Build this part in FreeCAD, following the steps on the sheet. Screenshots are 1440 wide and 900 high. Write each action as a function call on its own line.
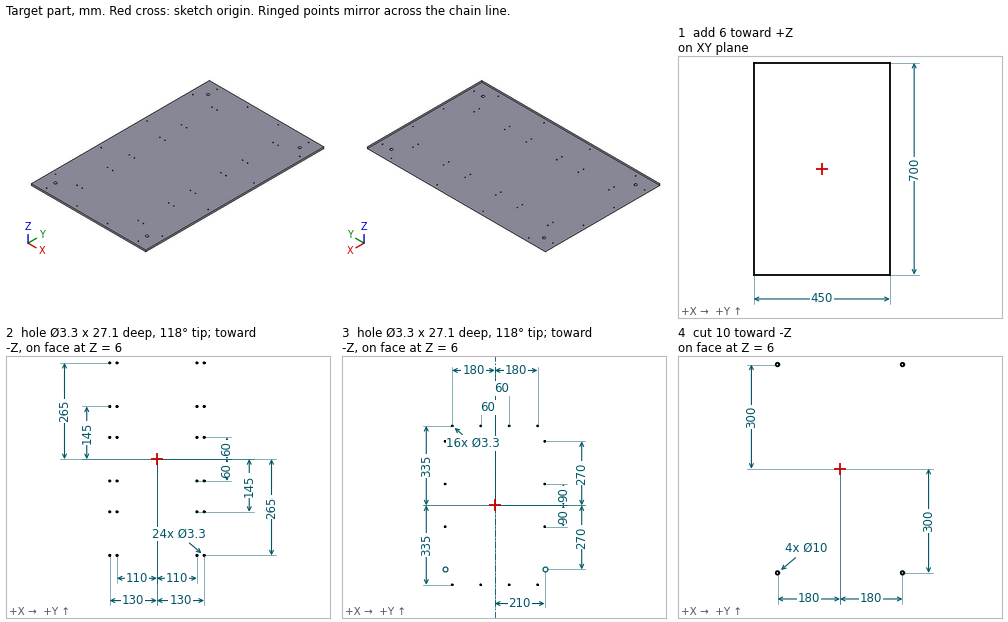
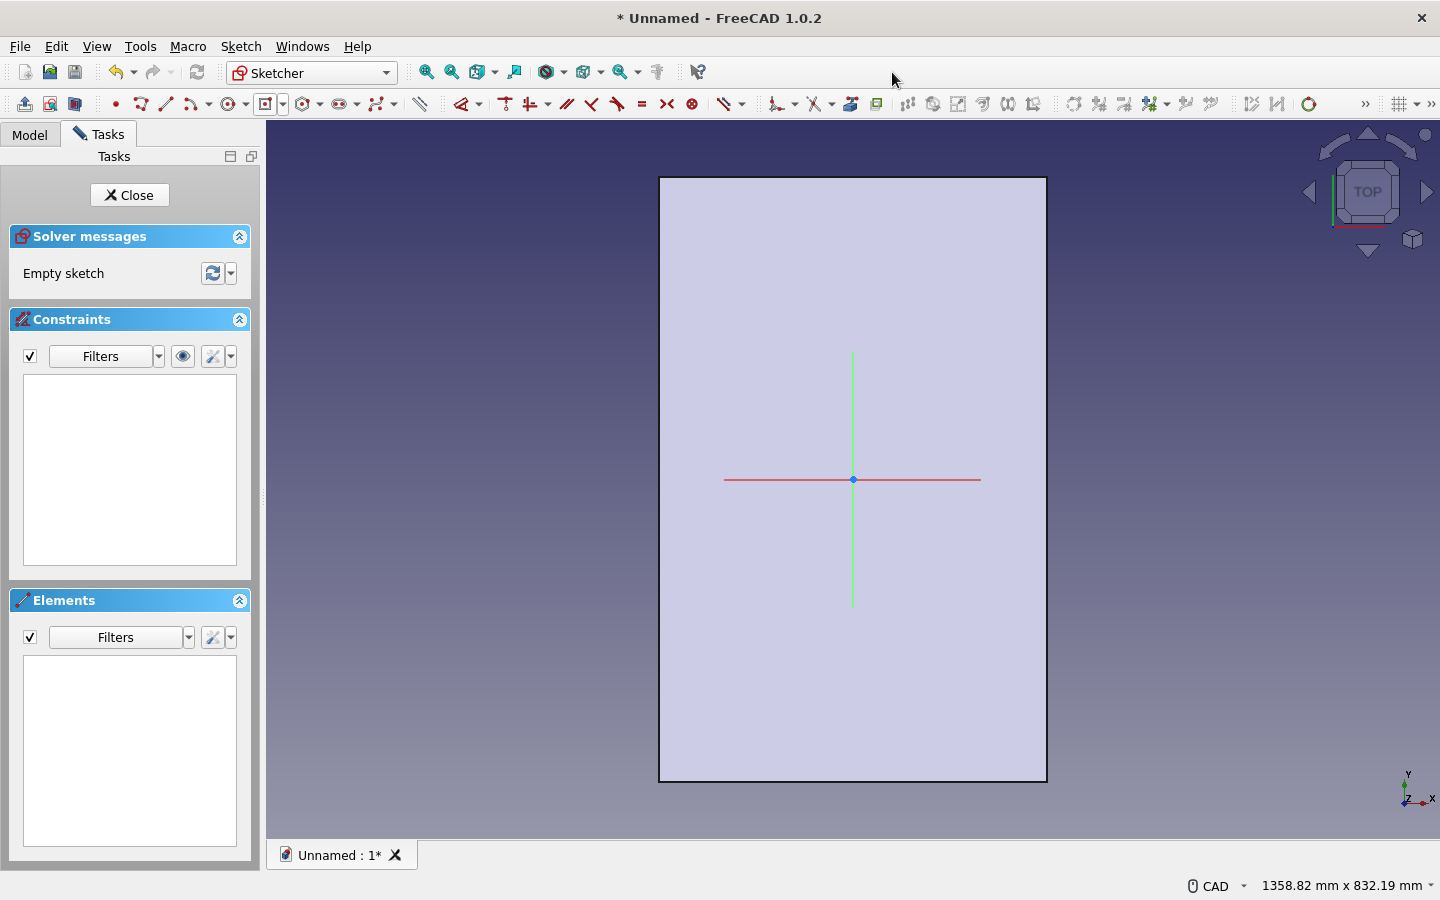
click(228, 104)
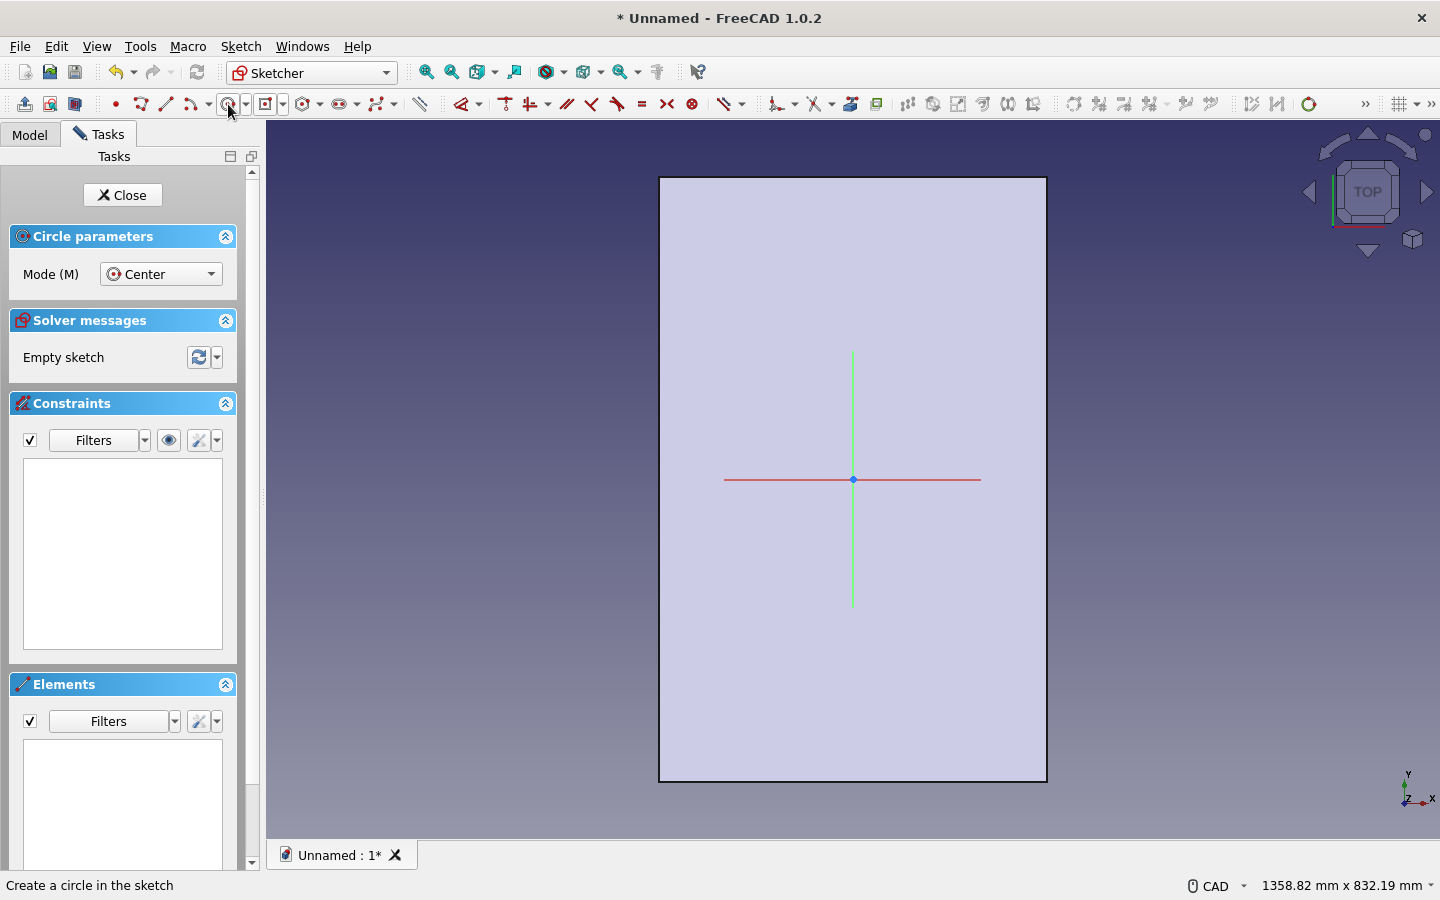
scroll(965, 708, up, 14)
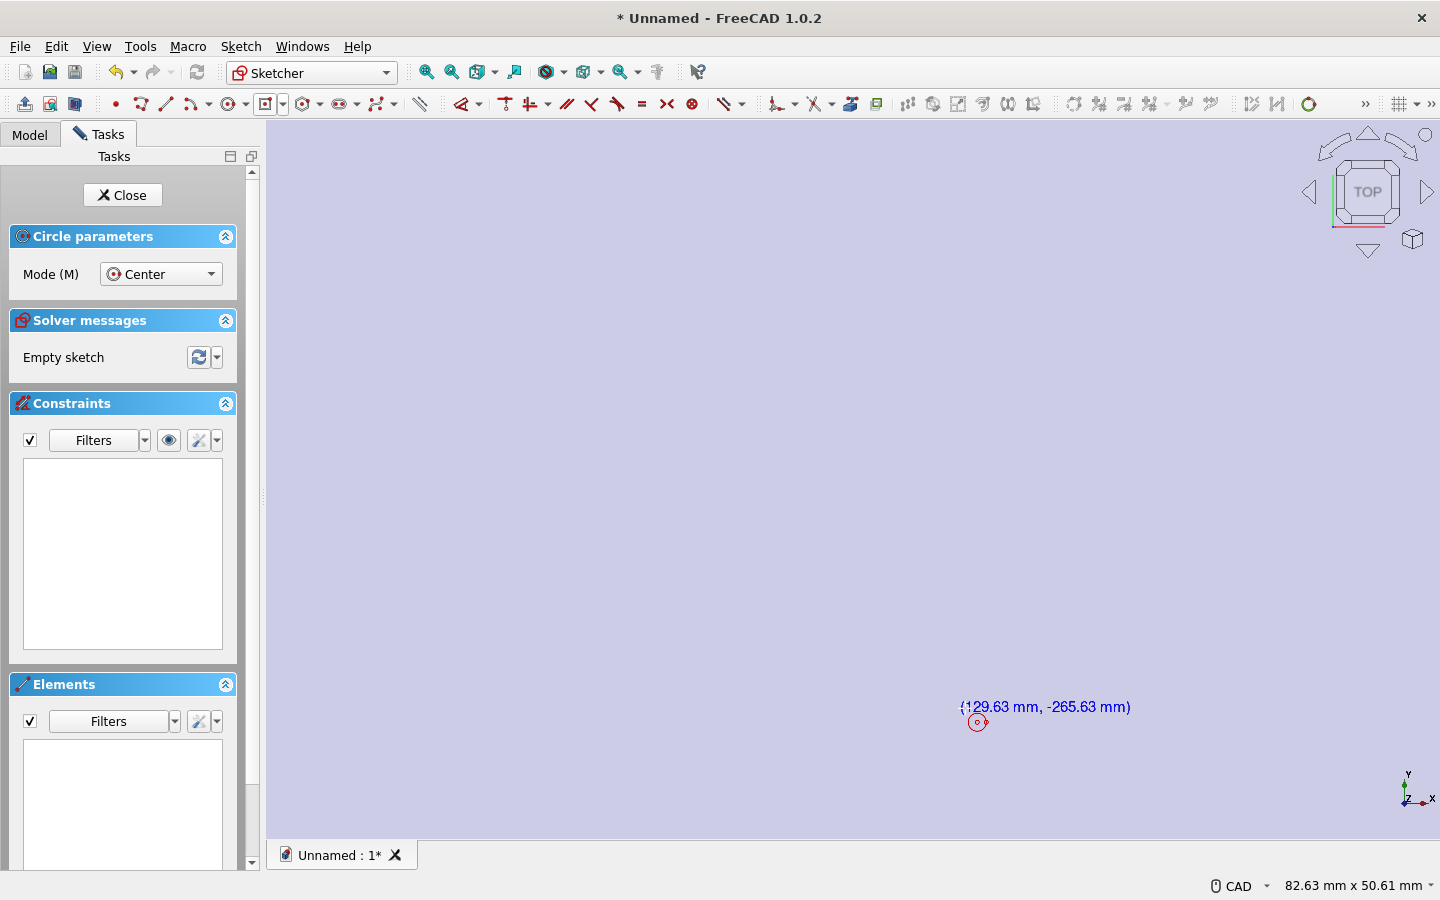
scroll(893, 709, down, 14)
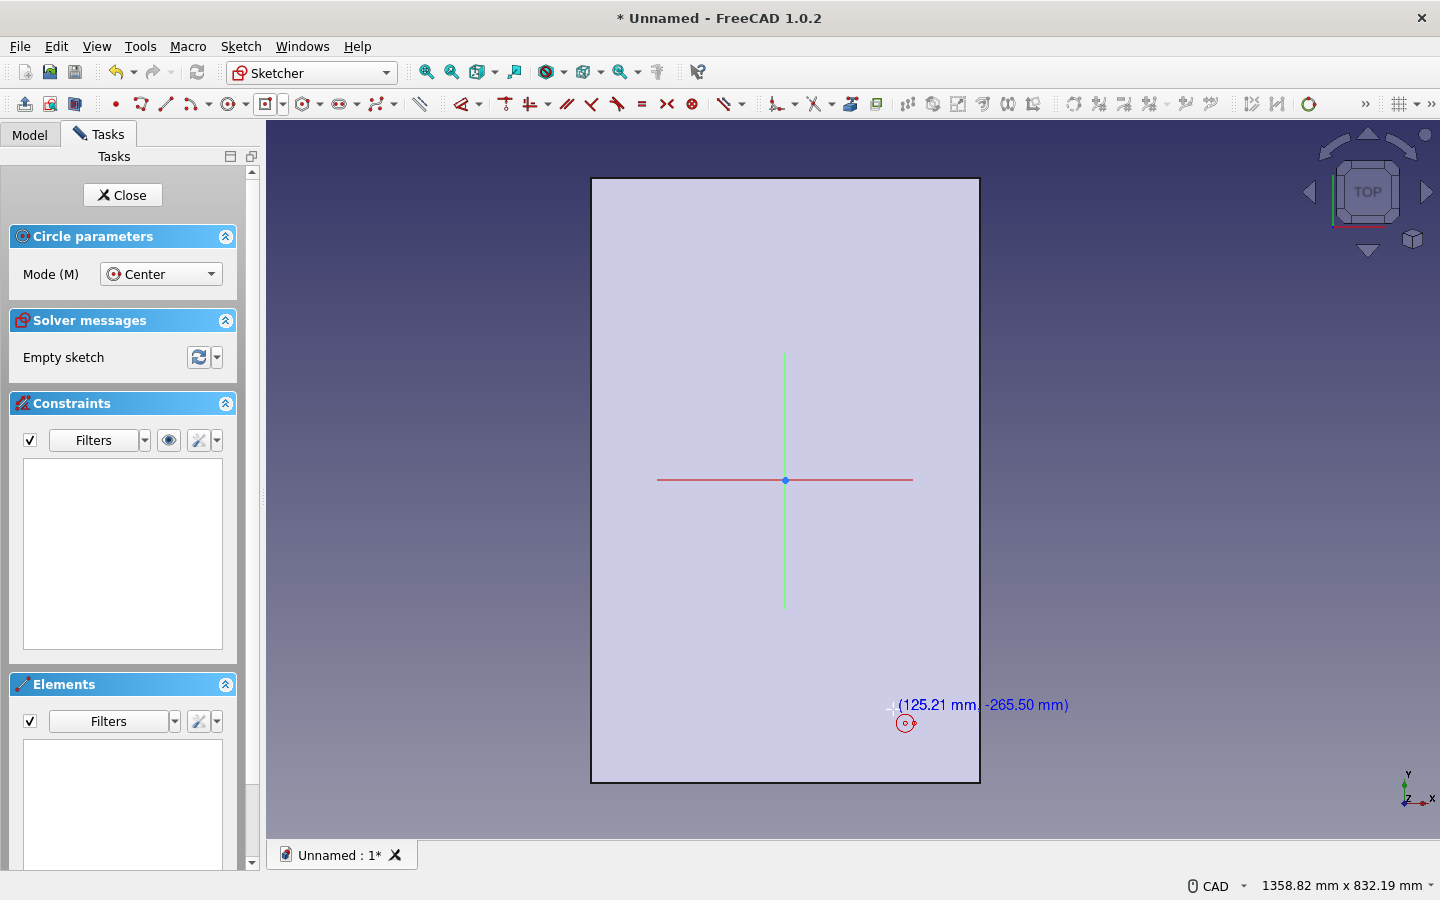
click(898, 709)
move(899, 708)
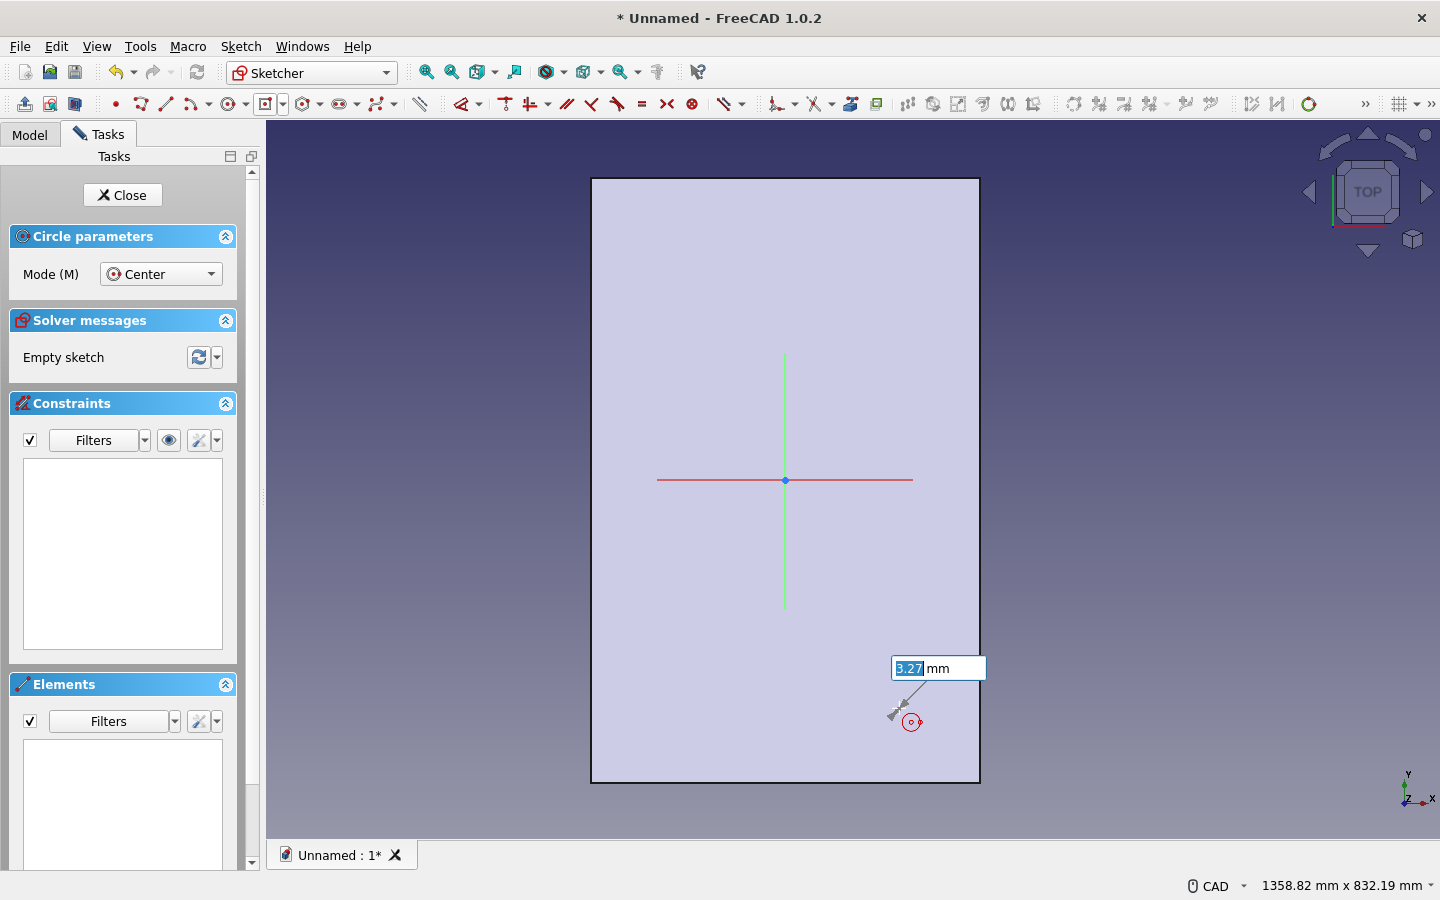
text(3.3)
key(Return)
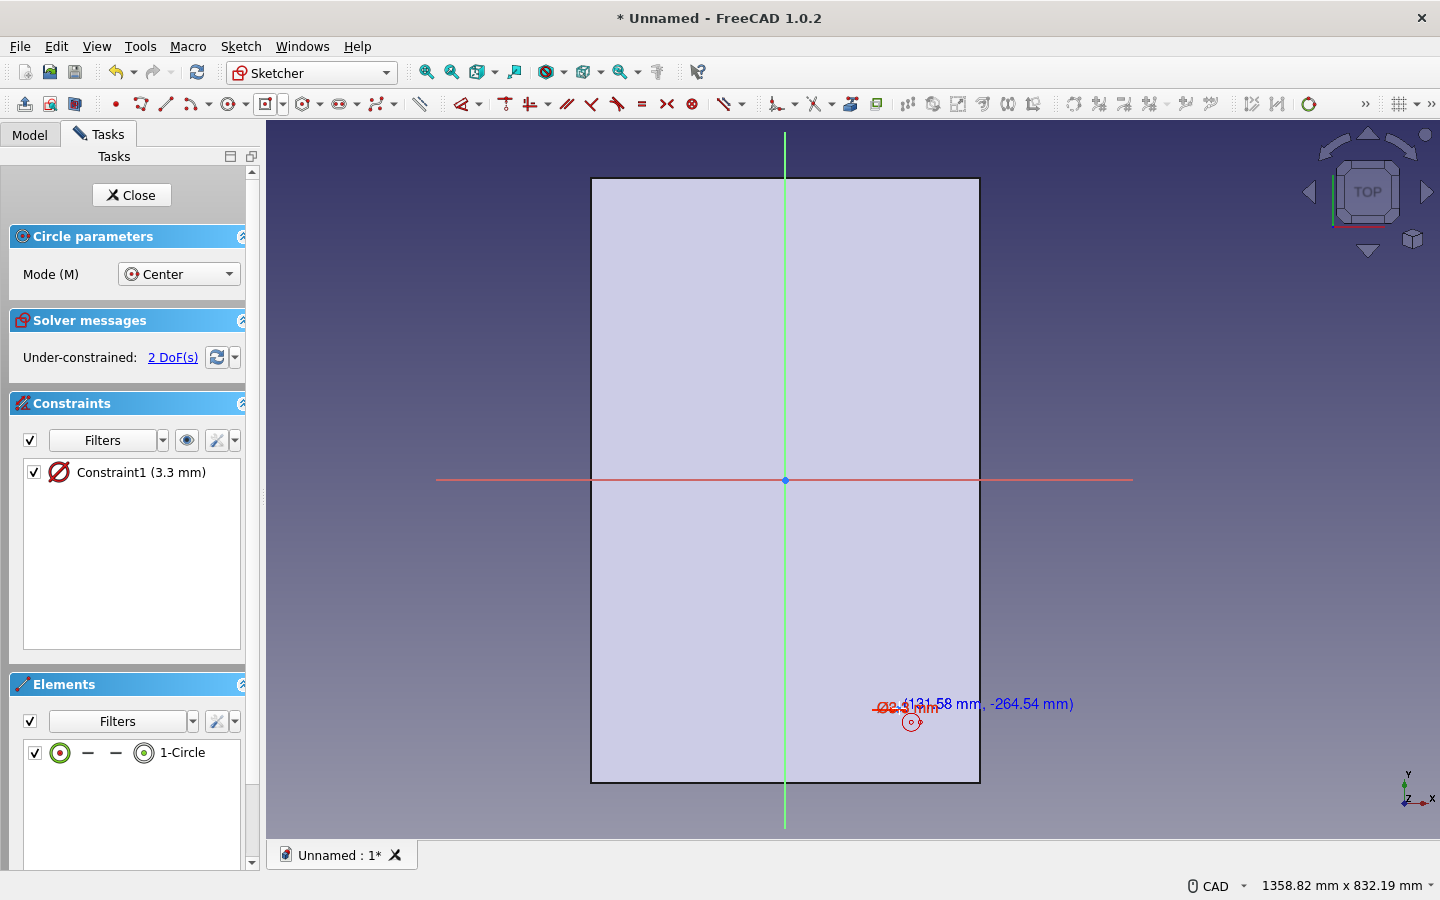
scroll(880, 709, up, 14)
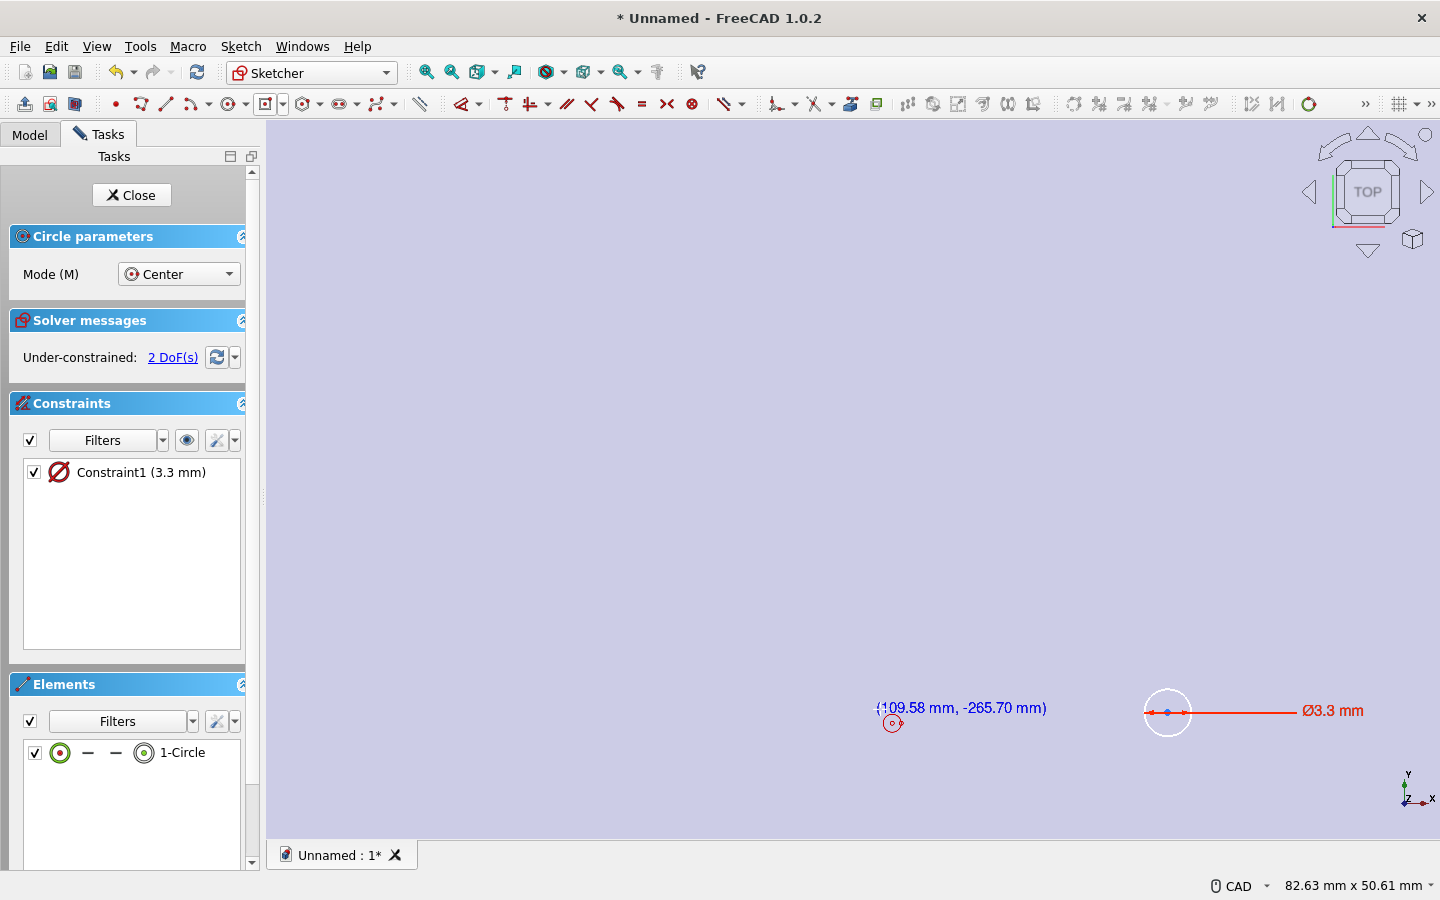
scroll(880, 709, down, 14)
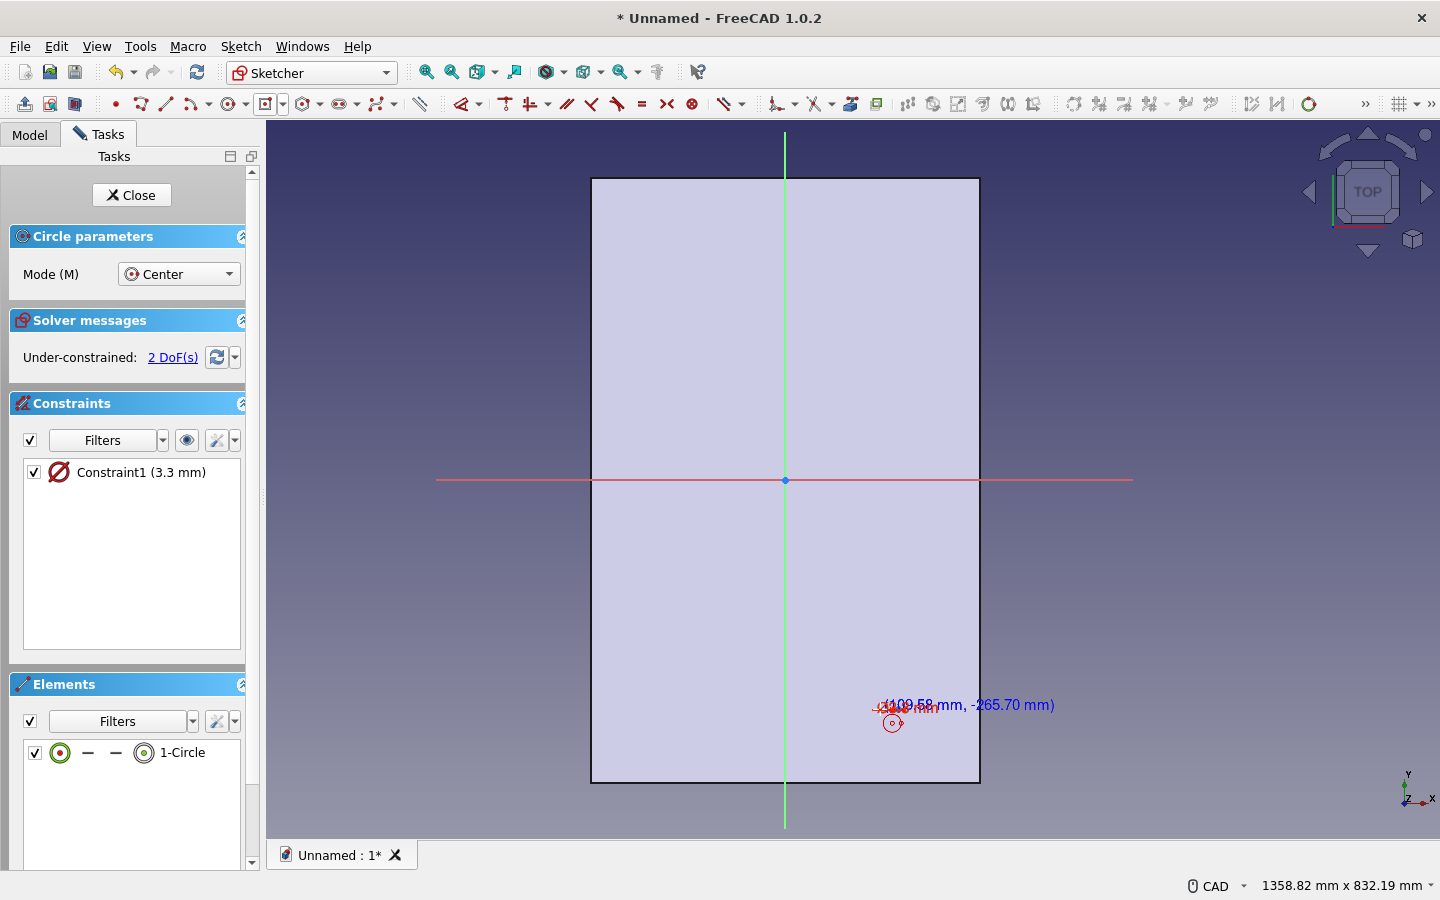
click(880, 709)
move(881, 708)